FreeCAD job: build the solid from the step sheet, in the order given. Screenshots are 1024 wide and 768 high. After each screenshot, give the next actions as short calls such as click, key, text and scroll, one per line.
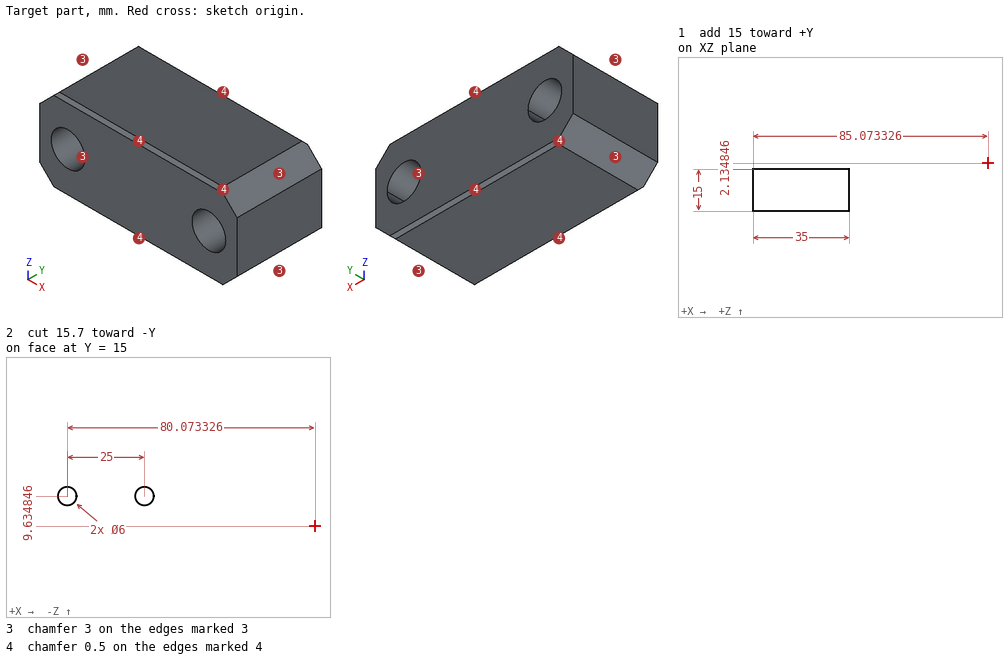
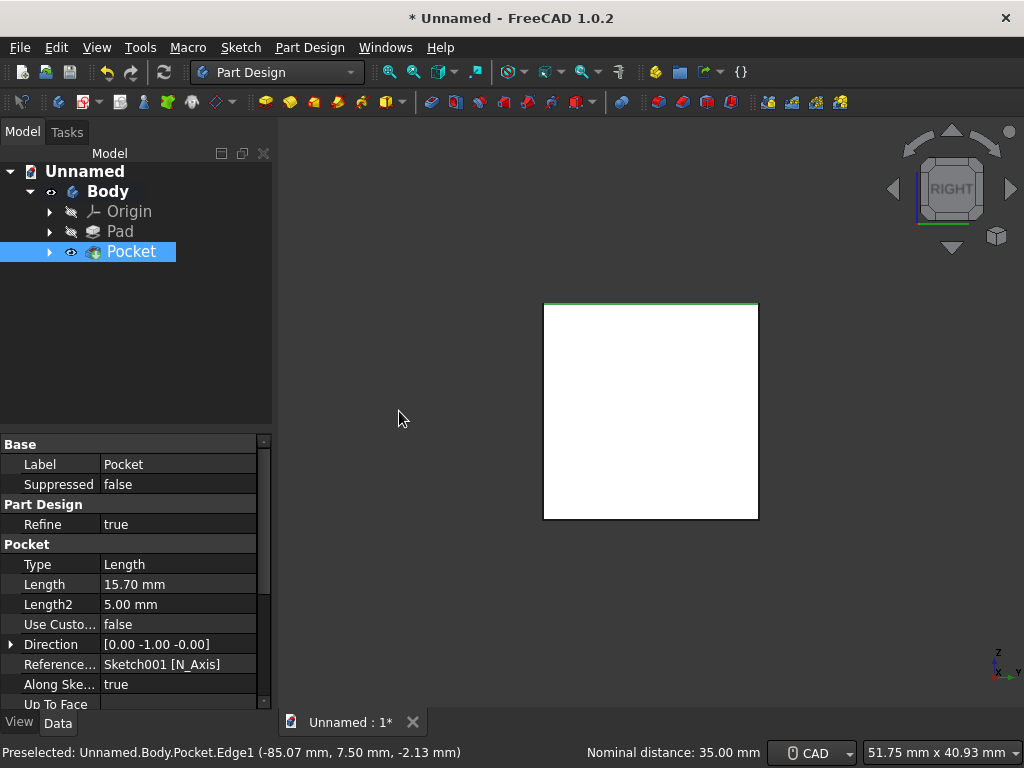
key(v)
key(f)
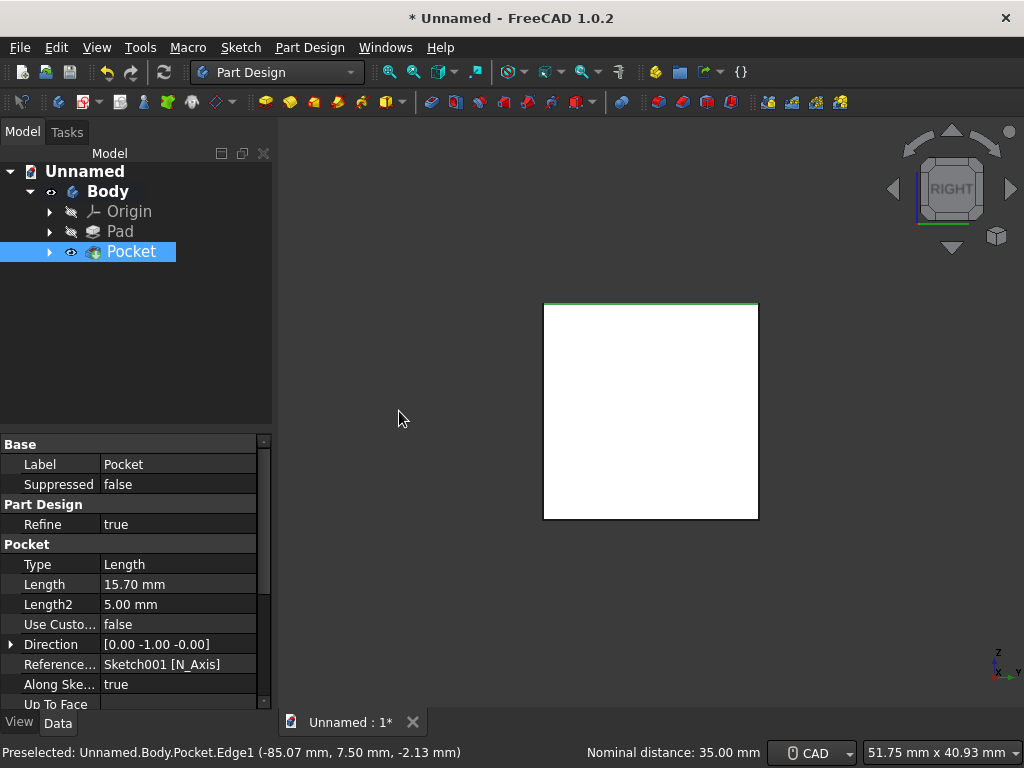
click(651, 519, ctrl)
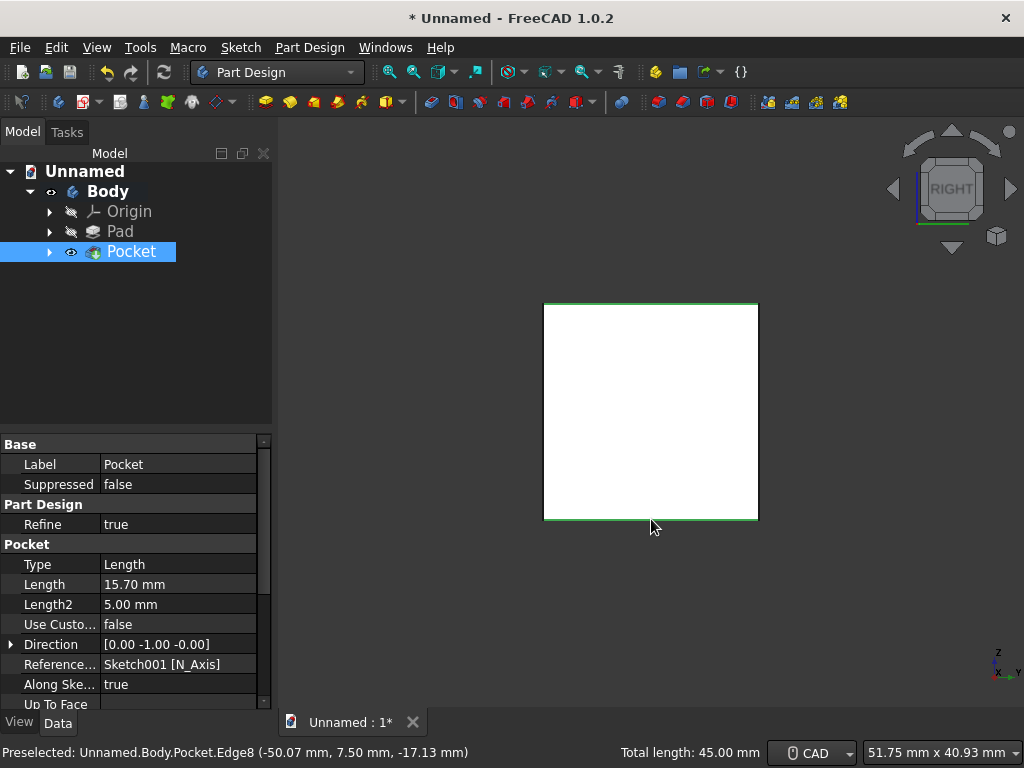
key(5)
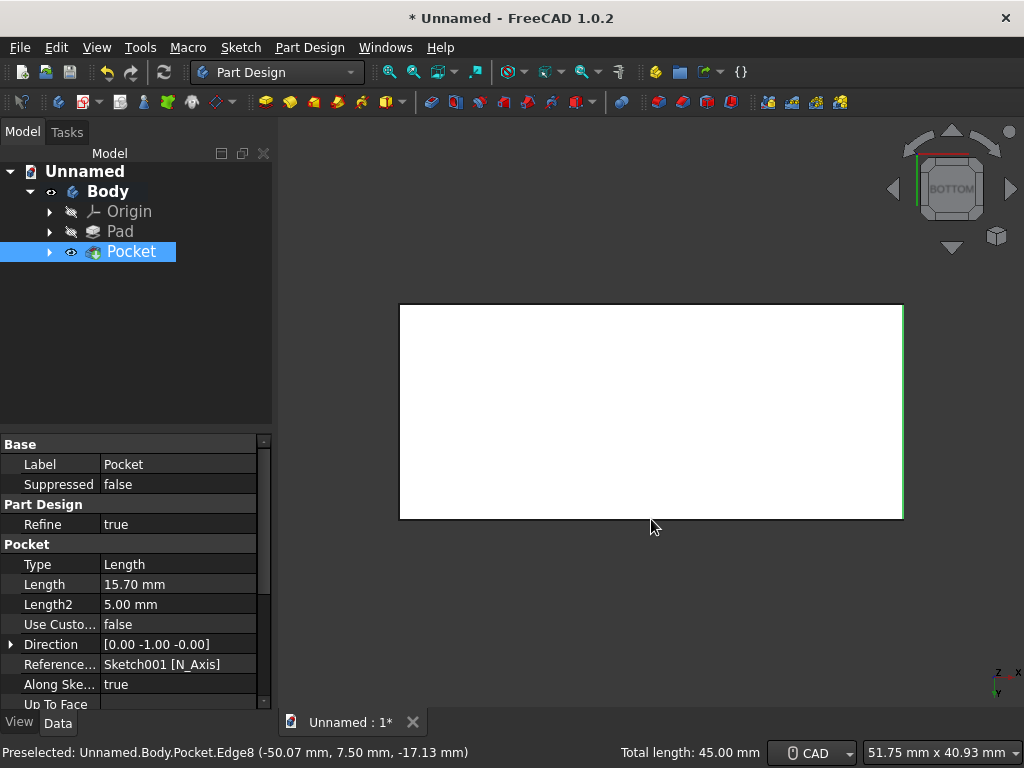
click(399, 411, ctrl)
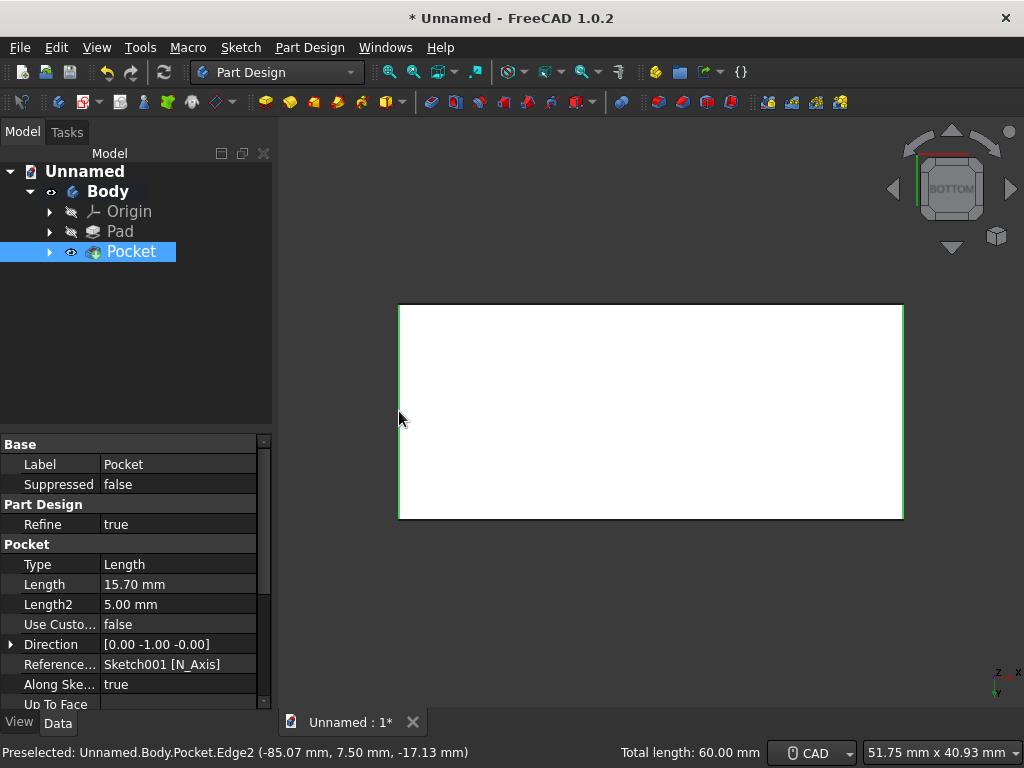
click(684, 102)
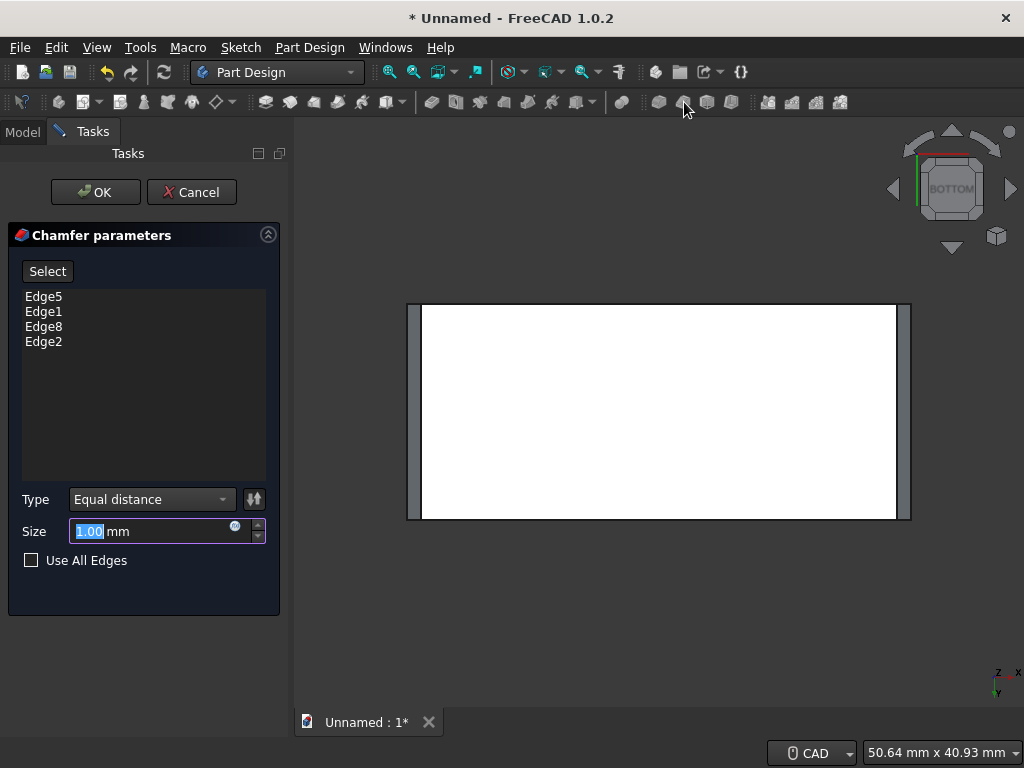
text(3)
key(Tab)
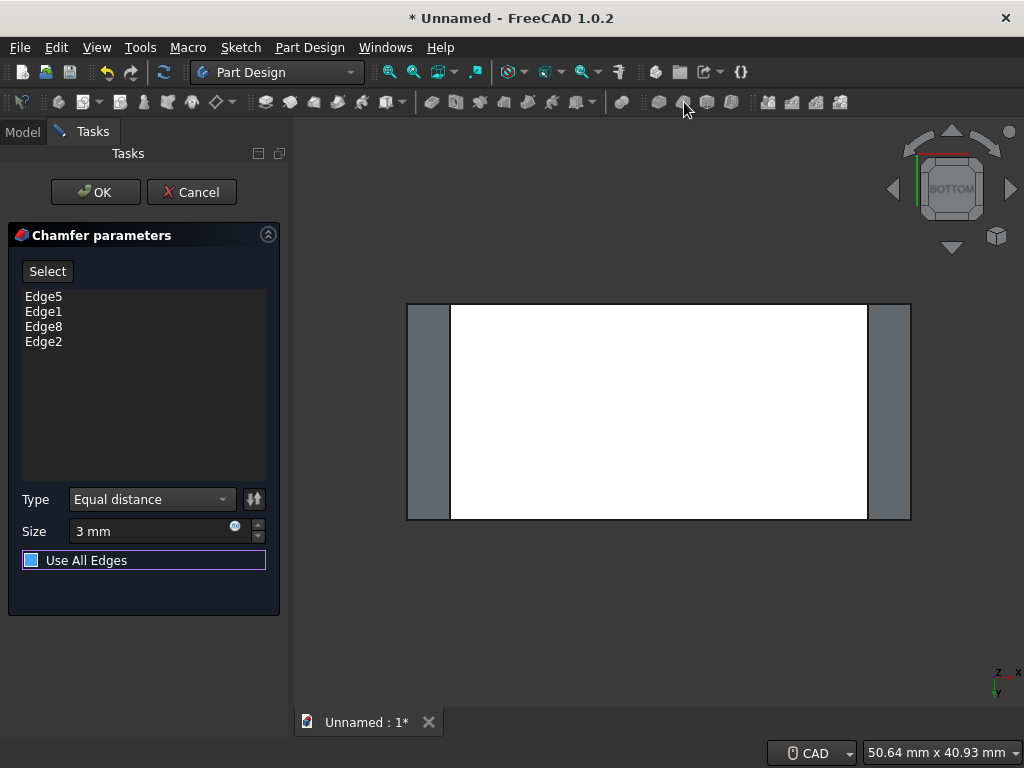
click(96, 192)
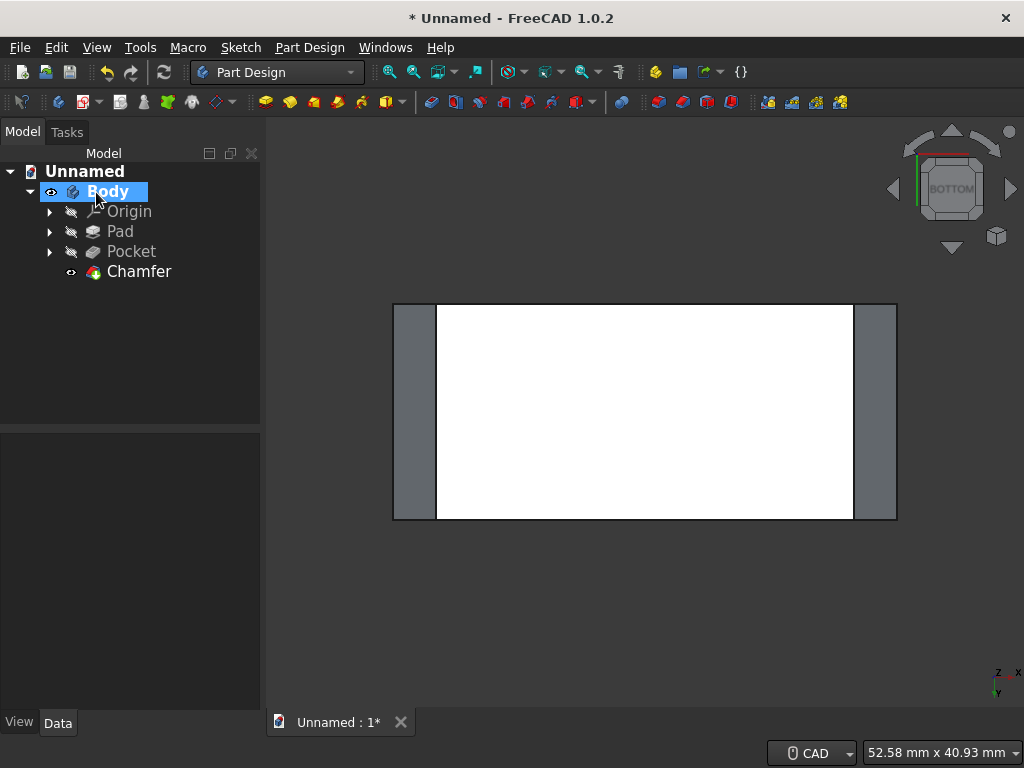
click(645, 303)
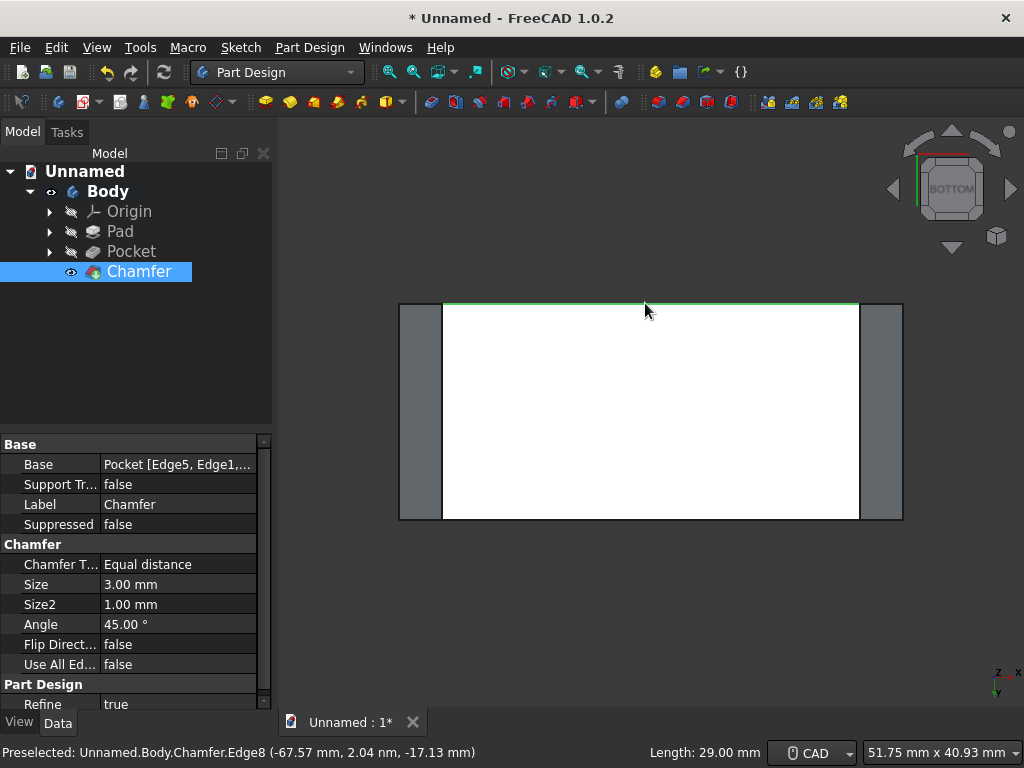
key(0)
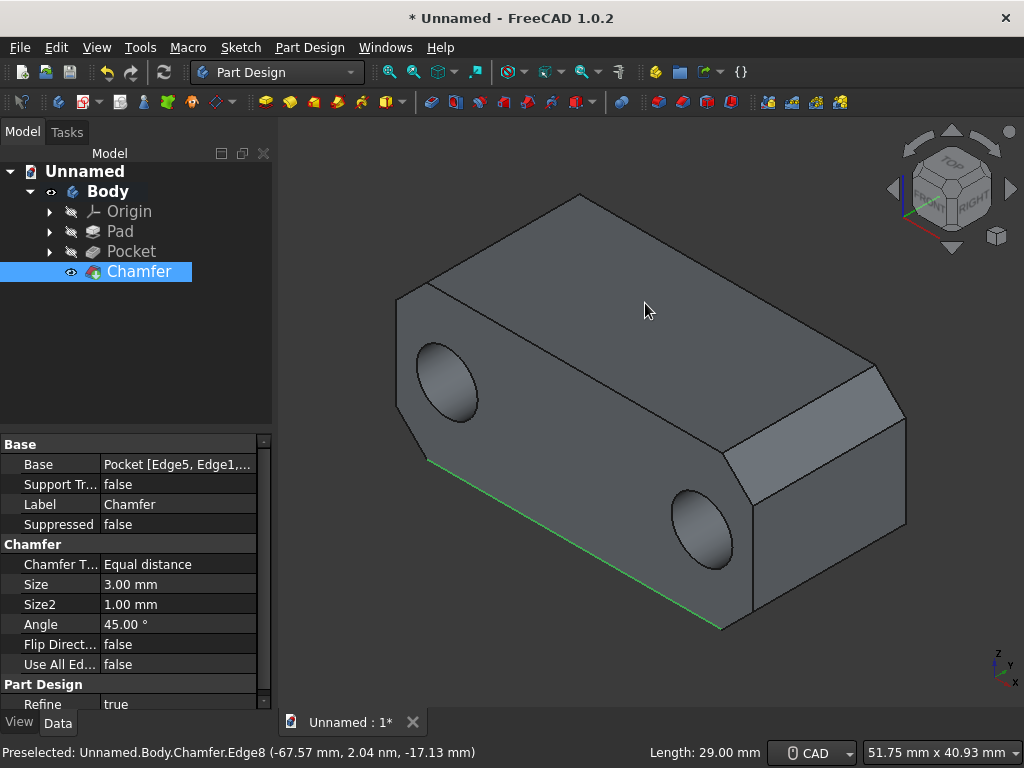
click(575, 367, ctrl)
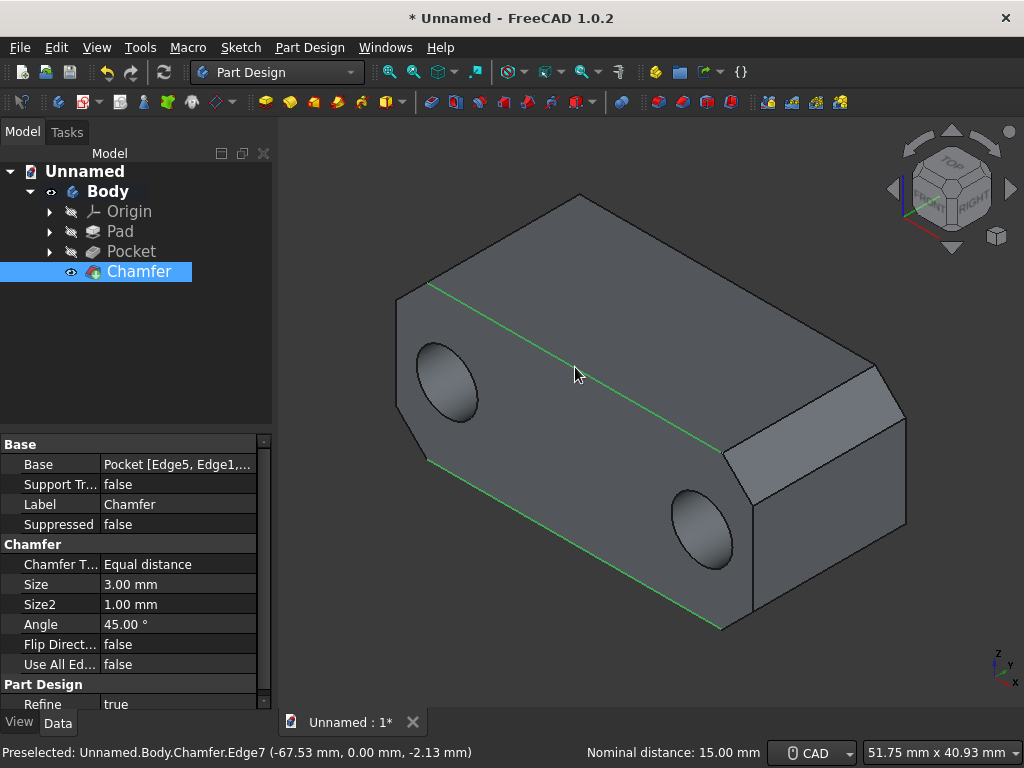
key(2)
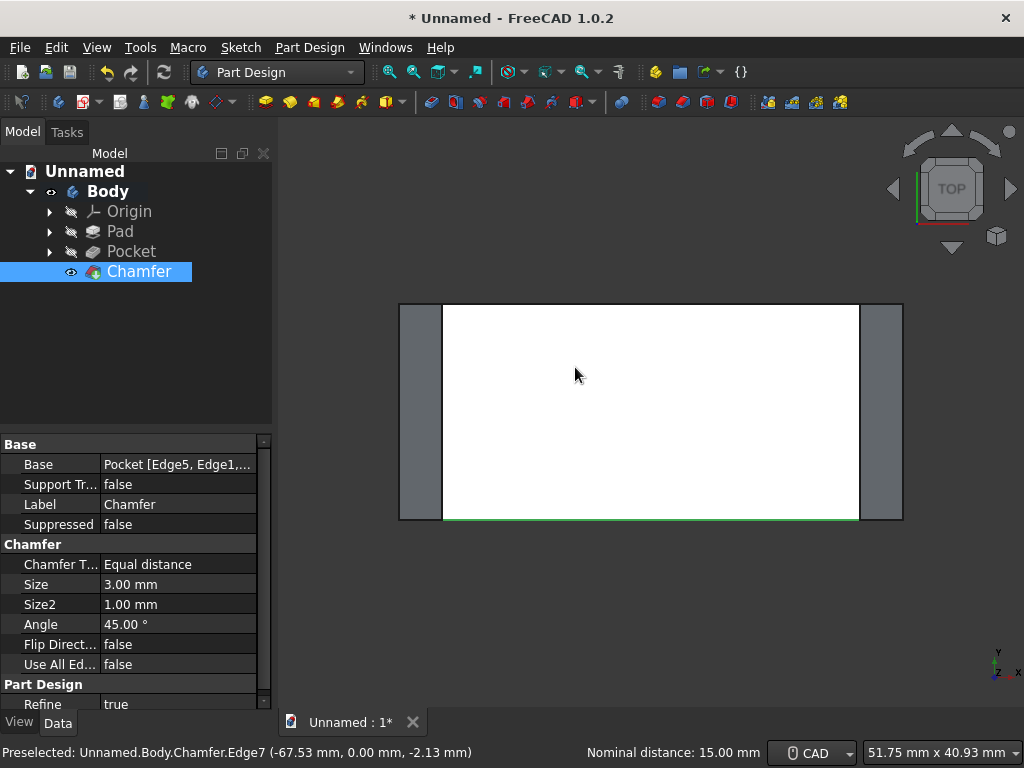
click(651, 303, ctrl)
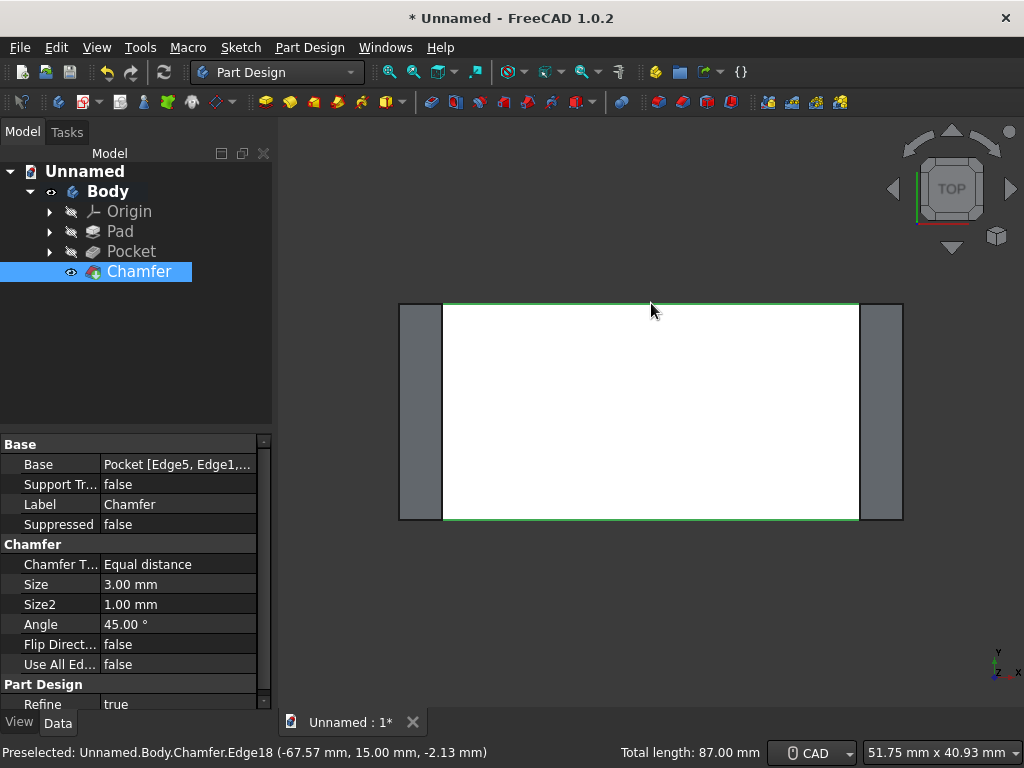
key(1)